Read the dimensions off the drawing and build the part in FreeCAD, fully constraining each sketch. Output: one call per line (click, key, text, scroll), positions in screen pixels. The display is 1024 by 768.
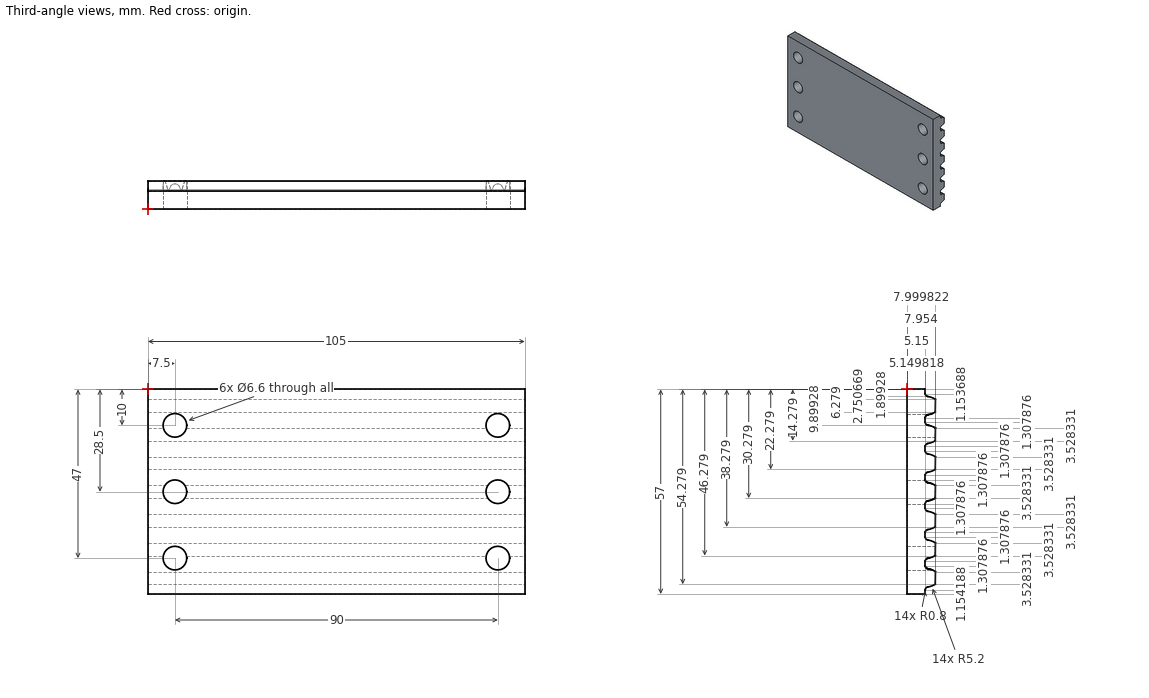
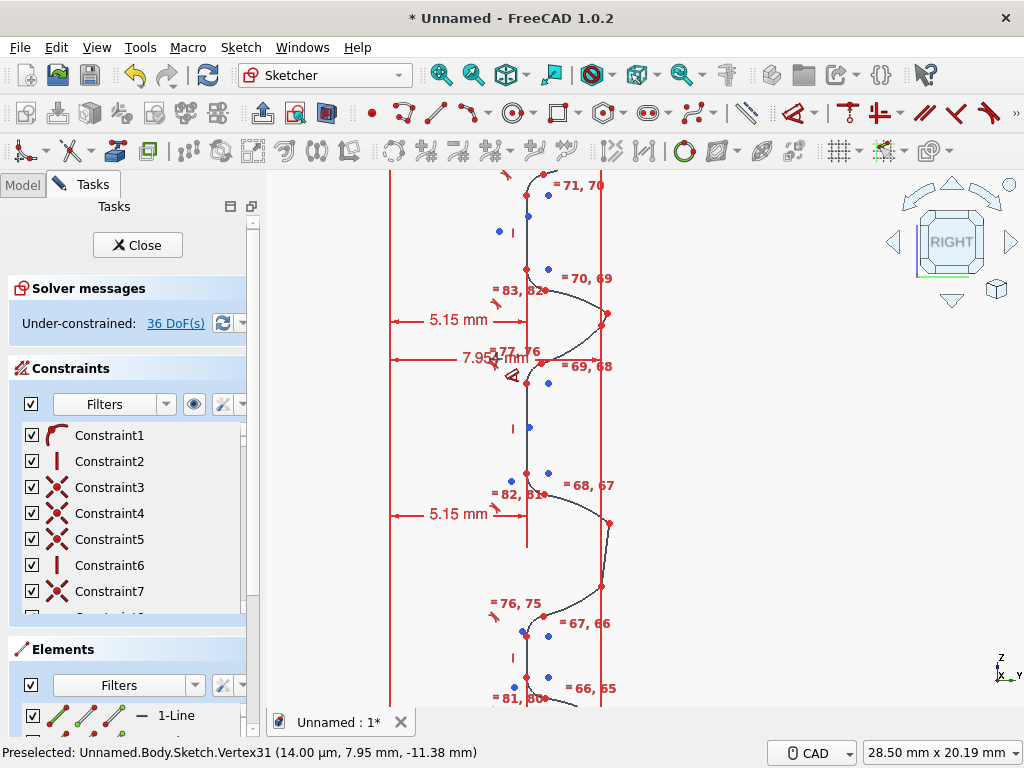
scroll(603, 326, down, 7)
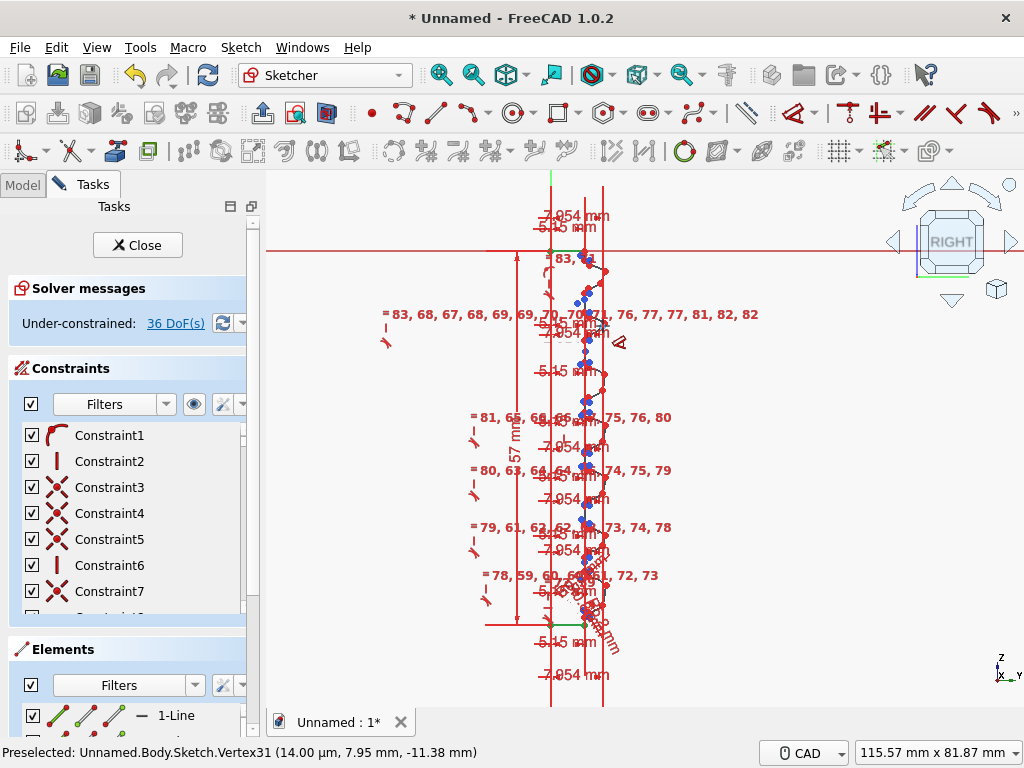
click(600, 283)
click(576, 389)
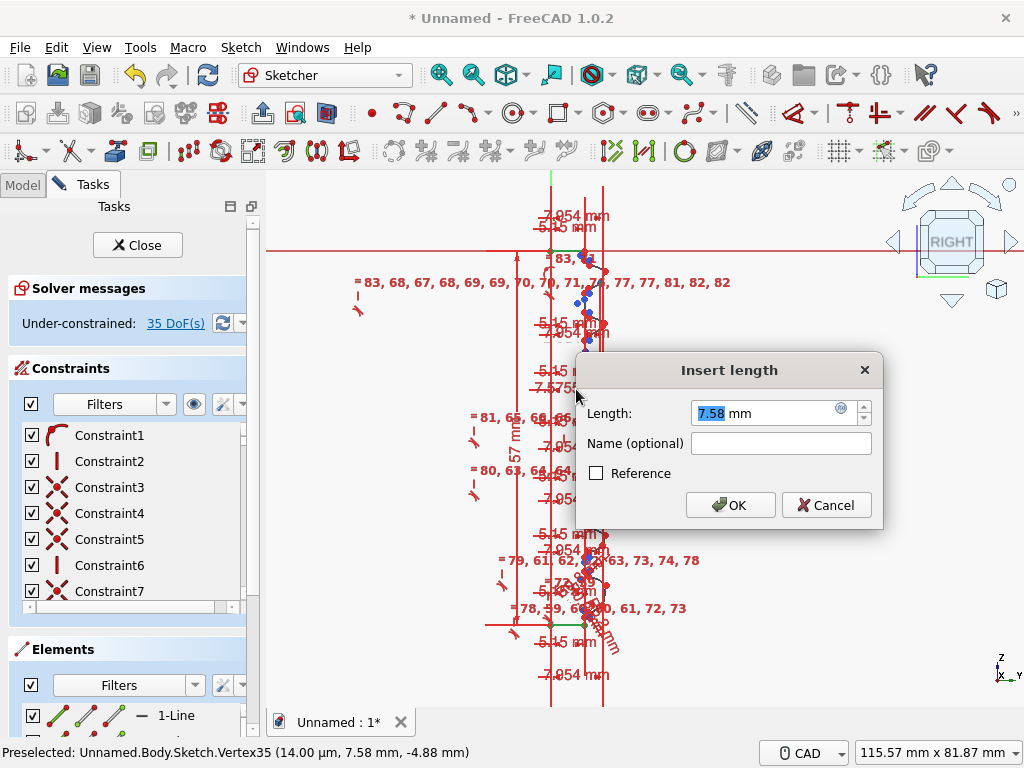
text(7.954)
key(Return)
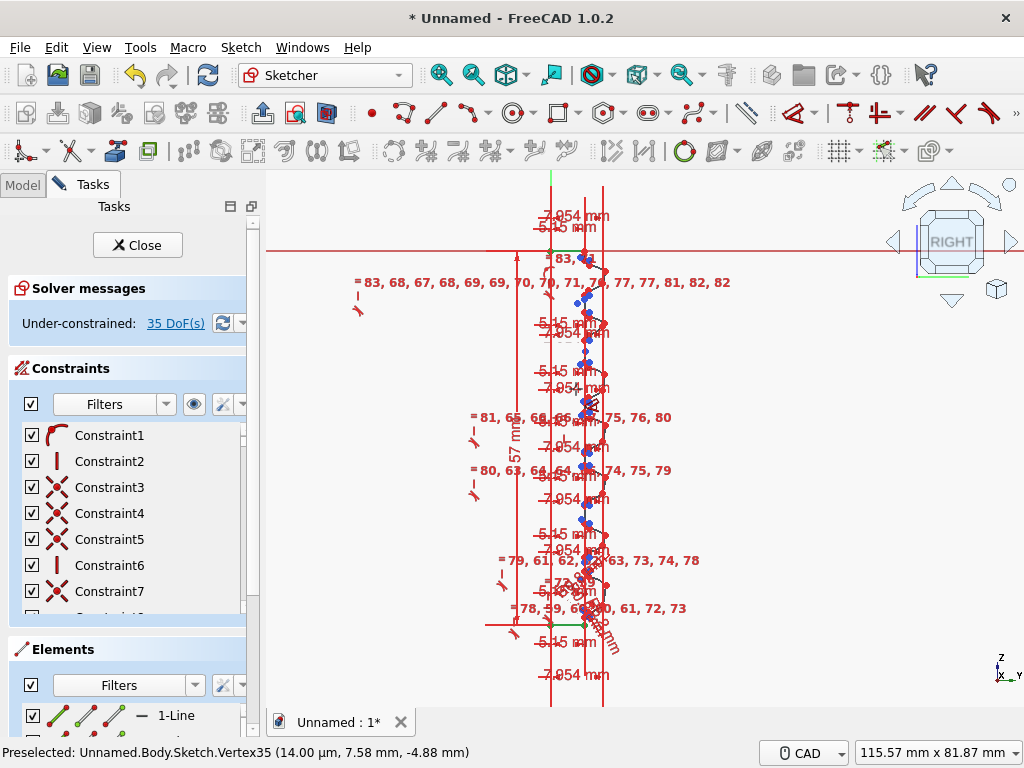
click(603, 283)
click(517, 267)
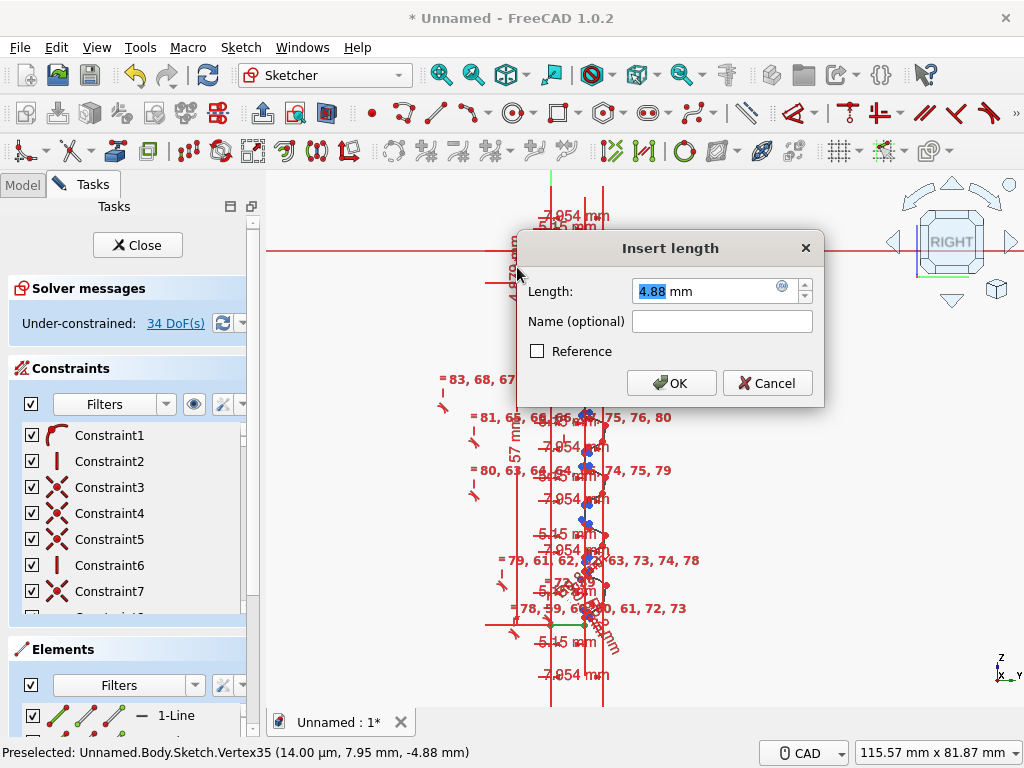
text(6.279)
key(Return)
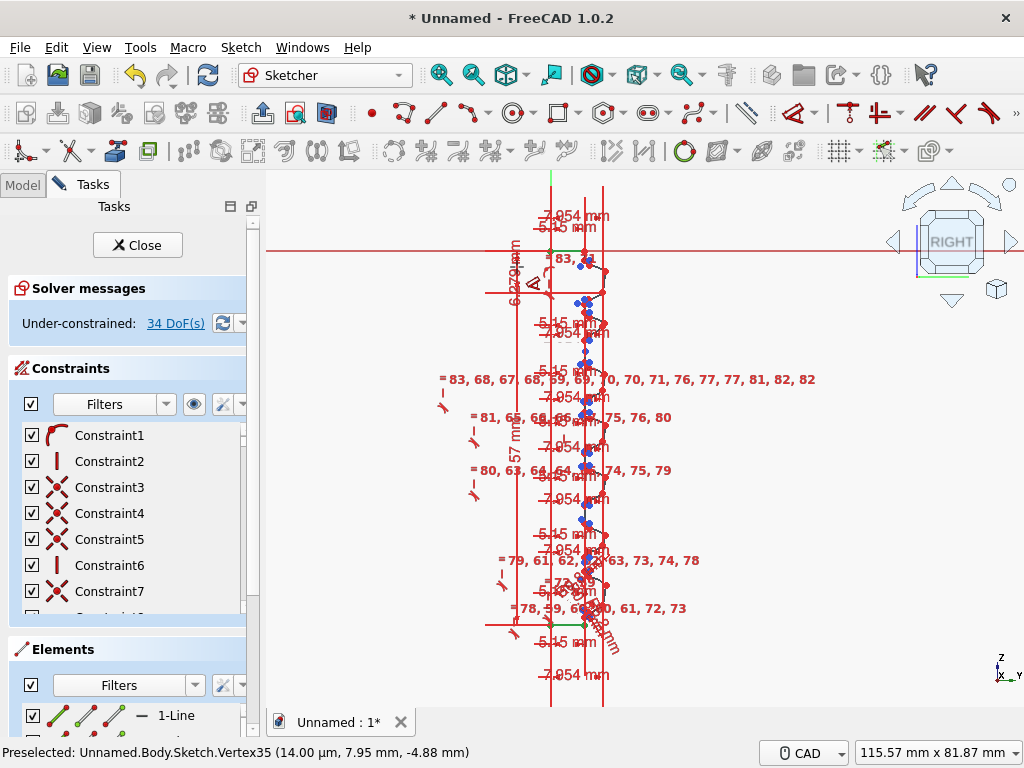
click(603, 605)
click(517, 304)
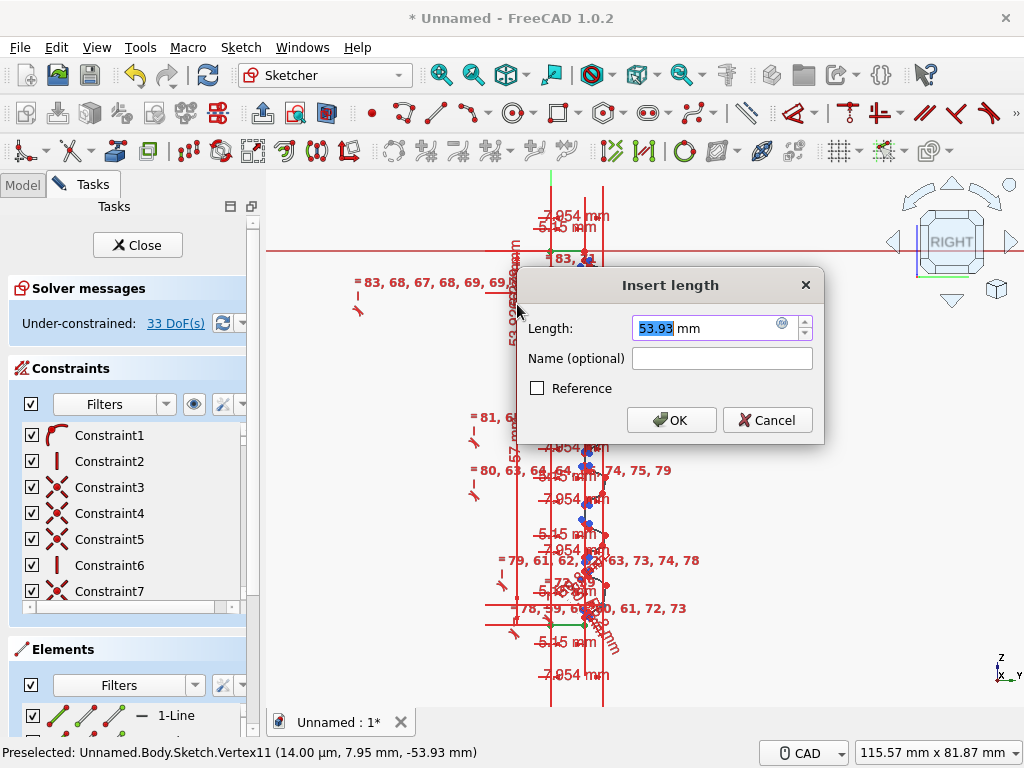
text(54.279)
key(Return)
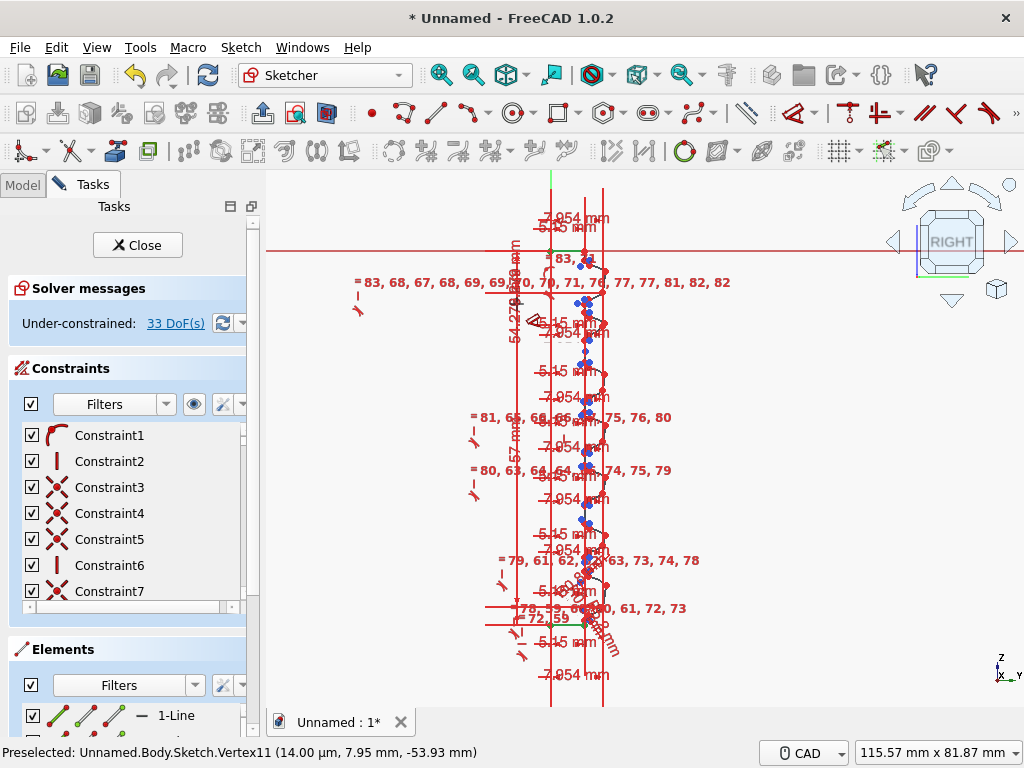
click(603, 546)
click(637, 296)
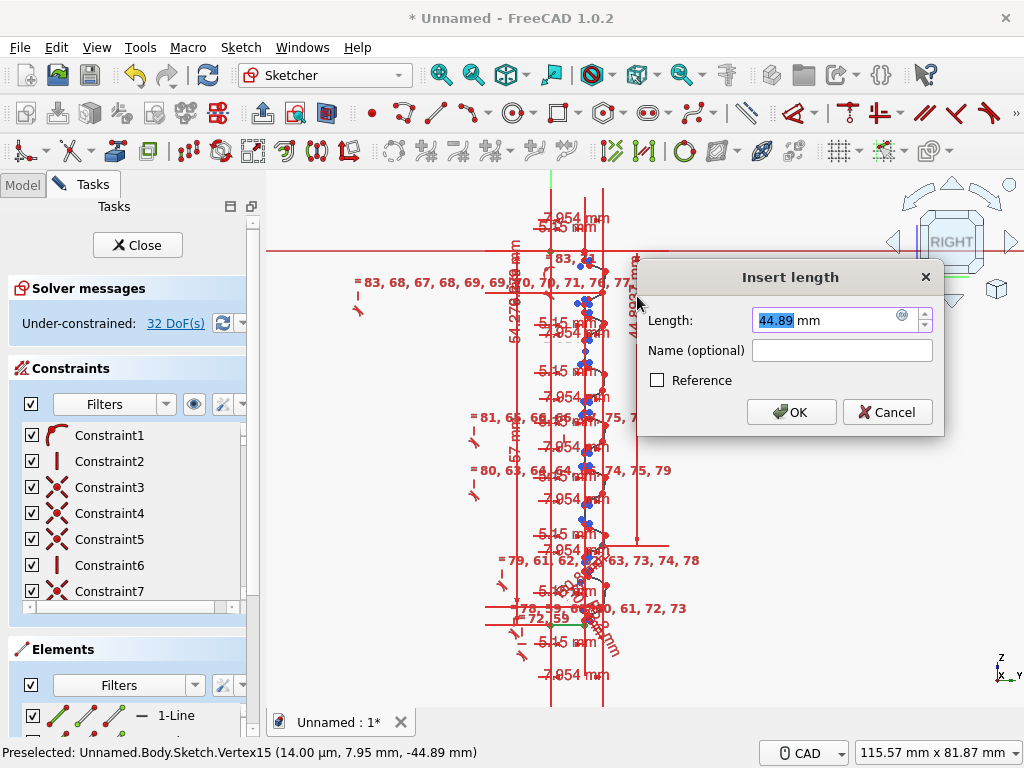
text(46.279)
key(Return)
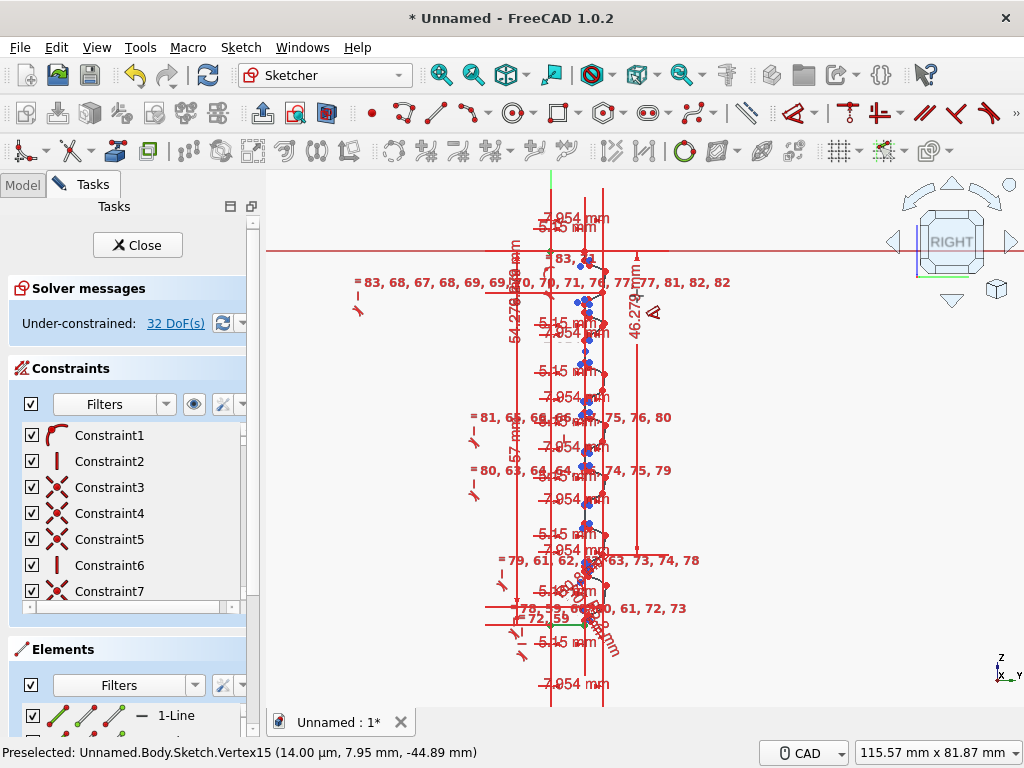
click(603, 493)
click(661, 372)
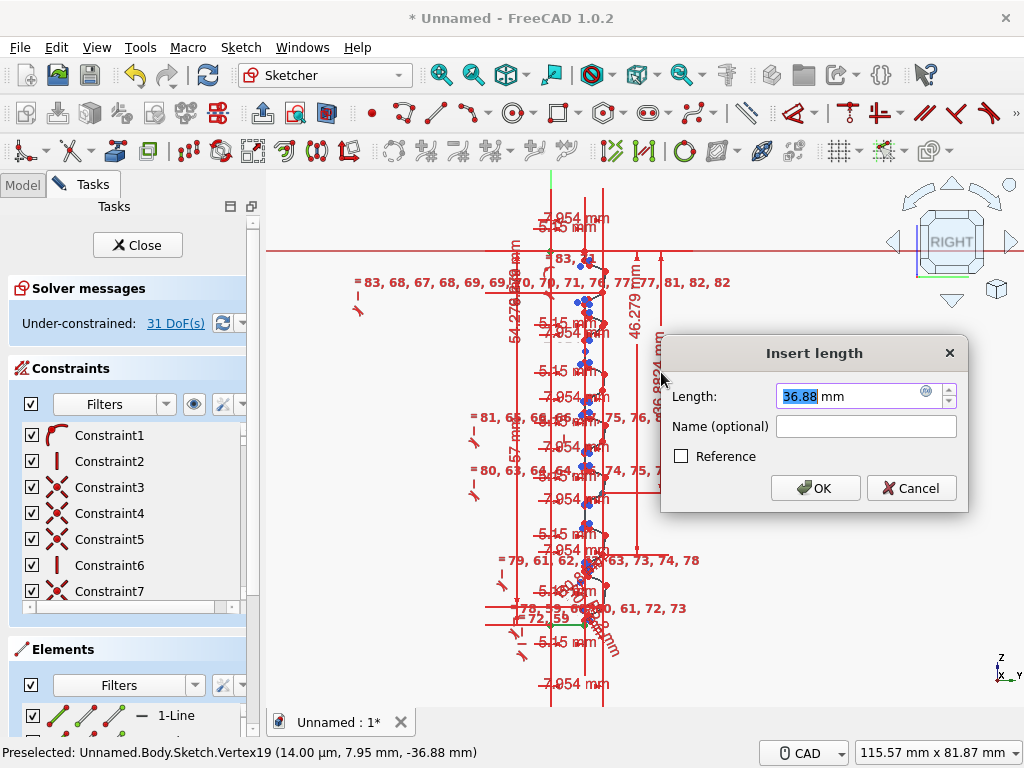
text(38.279)
key(Return)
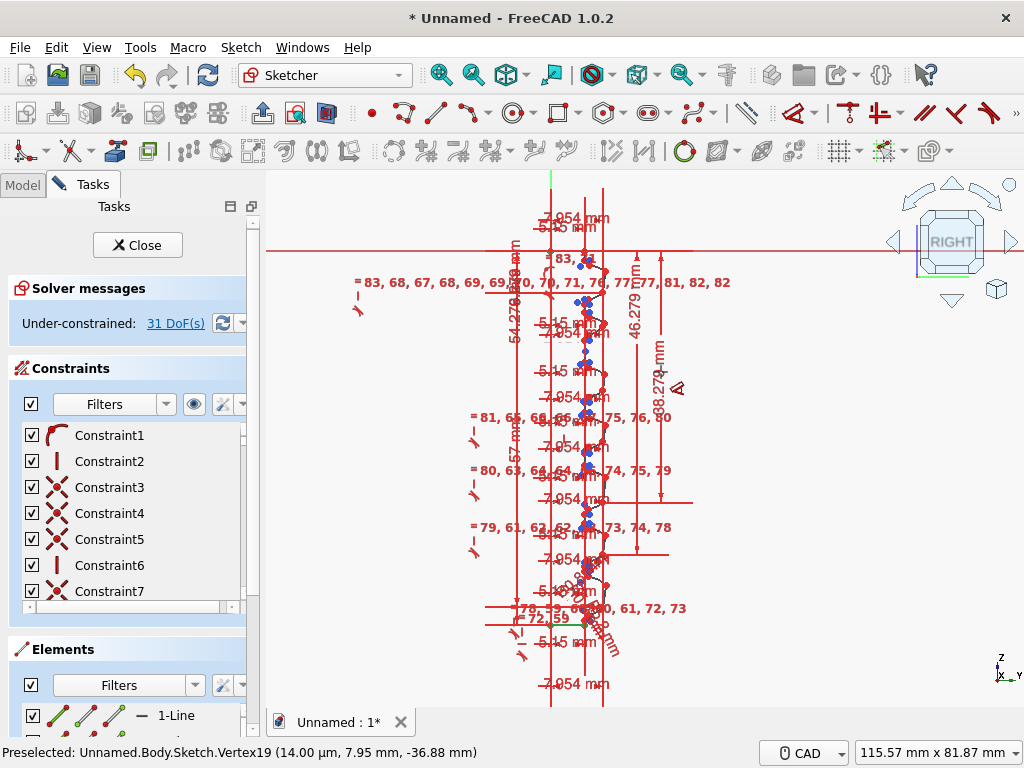
click(603, 442)
click(493, 347)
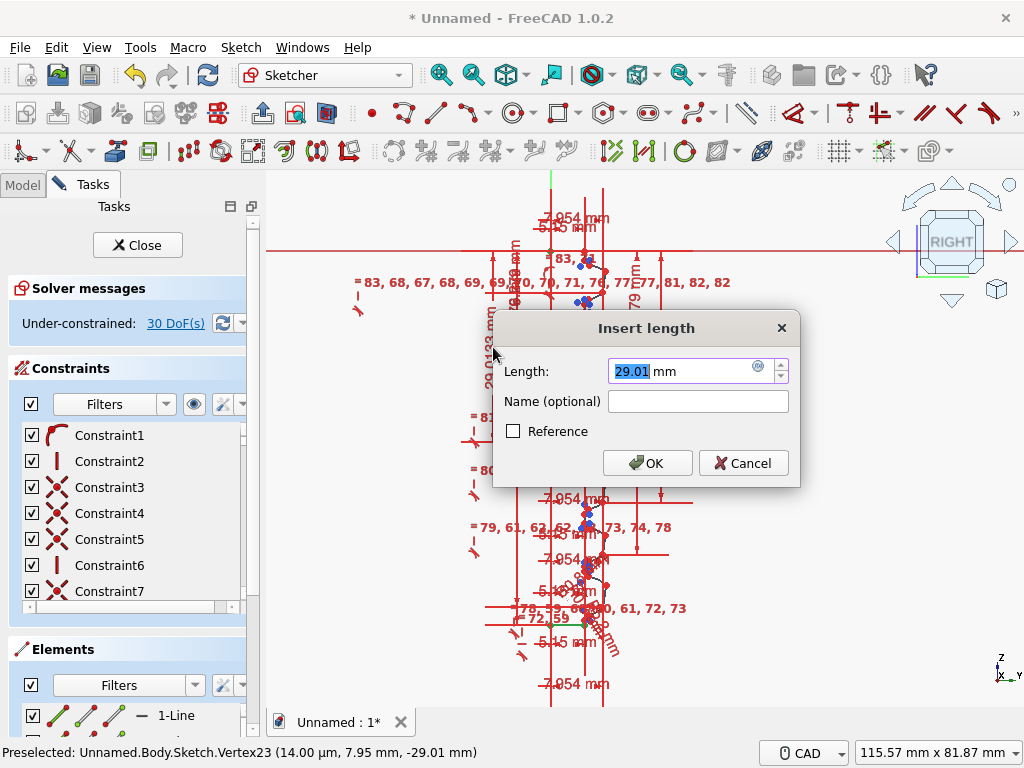
text(30.279)
key(Return)